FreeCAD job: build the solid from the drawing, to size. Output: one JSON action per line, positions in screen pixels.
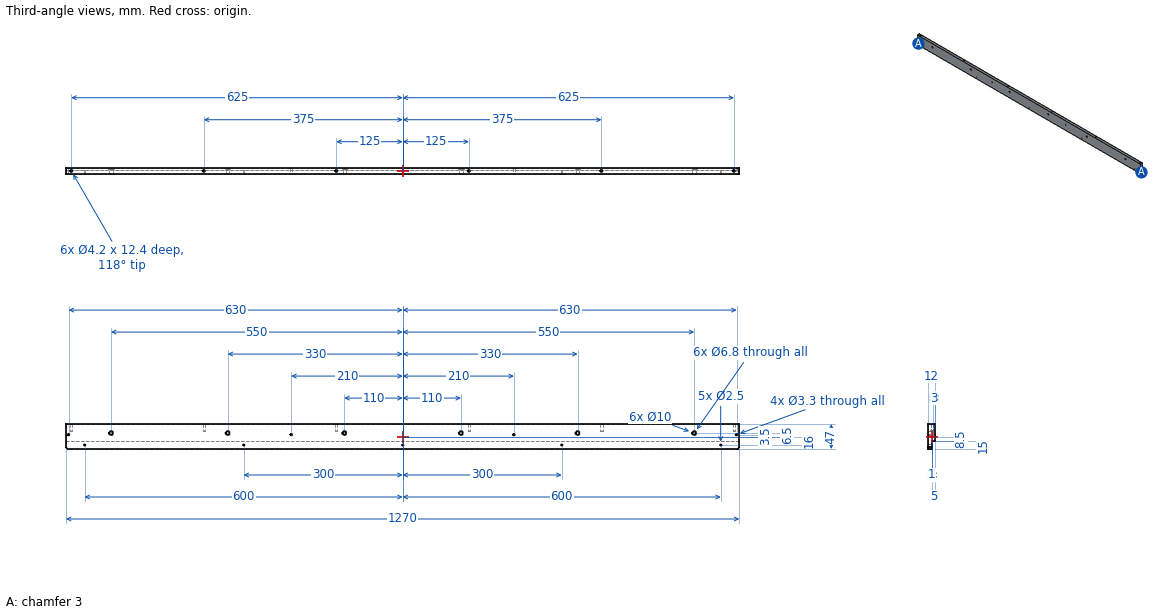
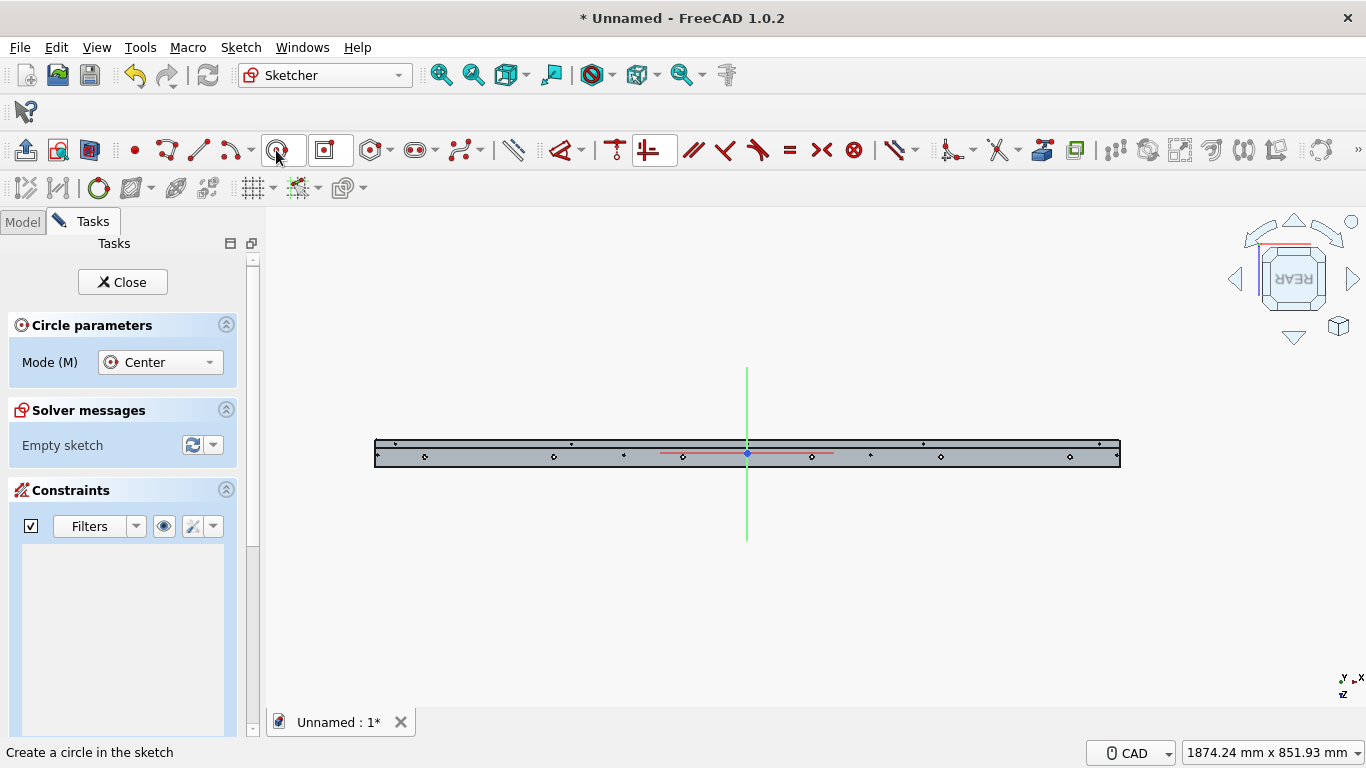
{"action": "scroll", "coordinate": [1070, 457], "scroll_direction": "up", "scroll_amount": 11}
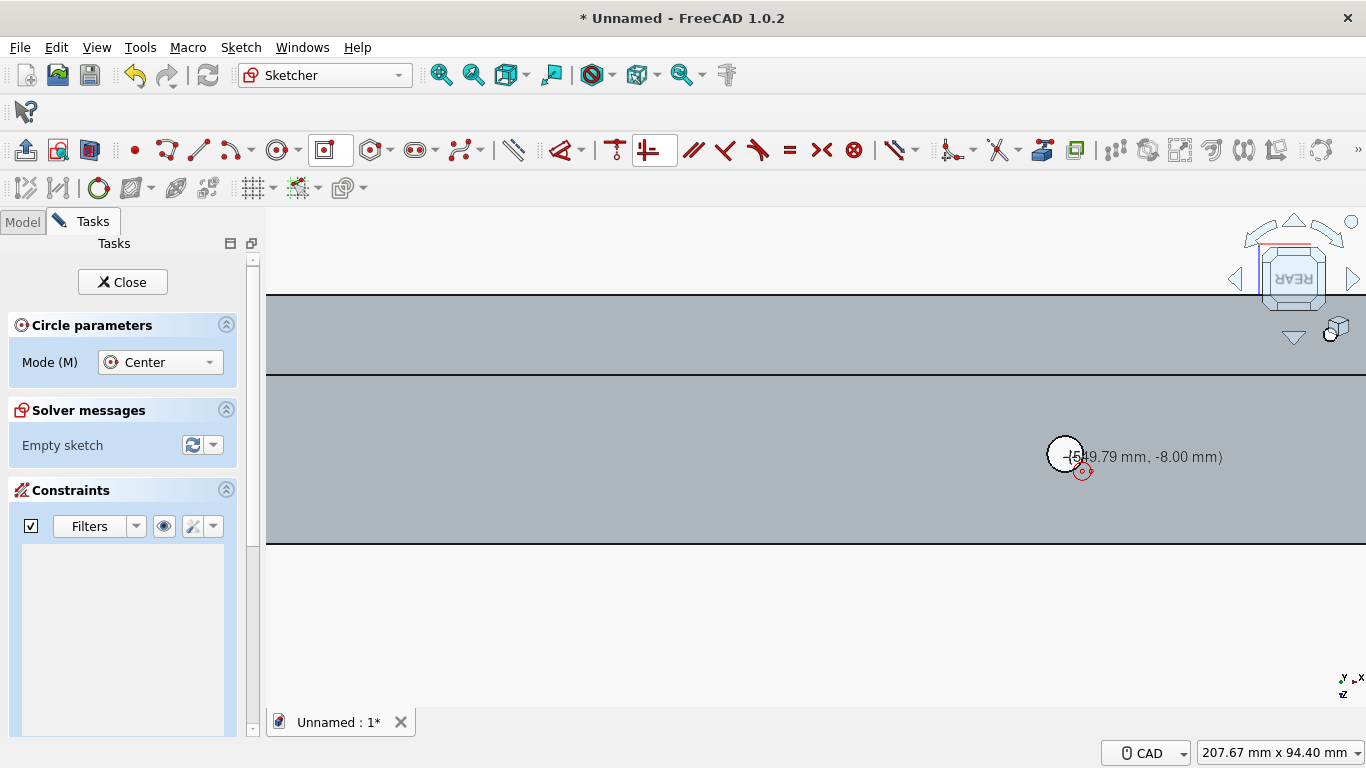
{"action": "left_click", "coordinate": [1065, 454]}
{"action": "mouse_move", "coordinate": [1084, 435]}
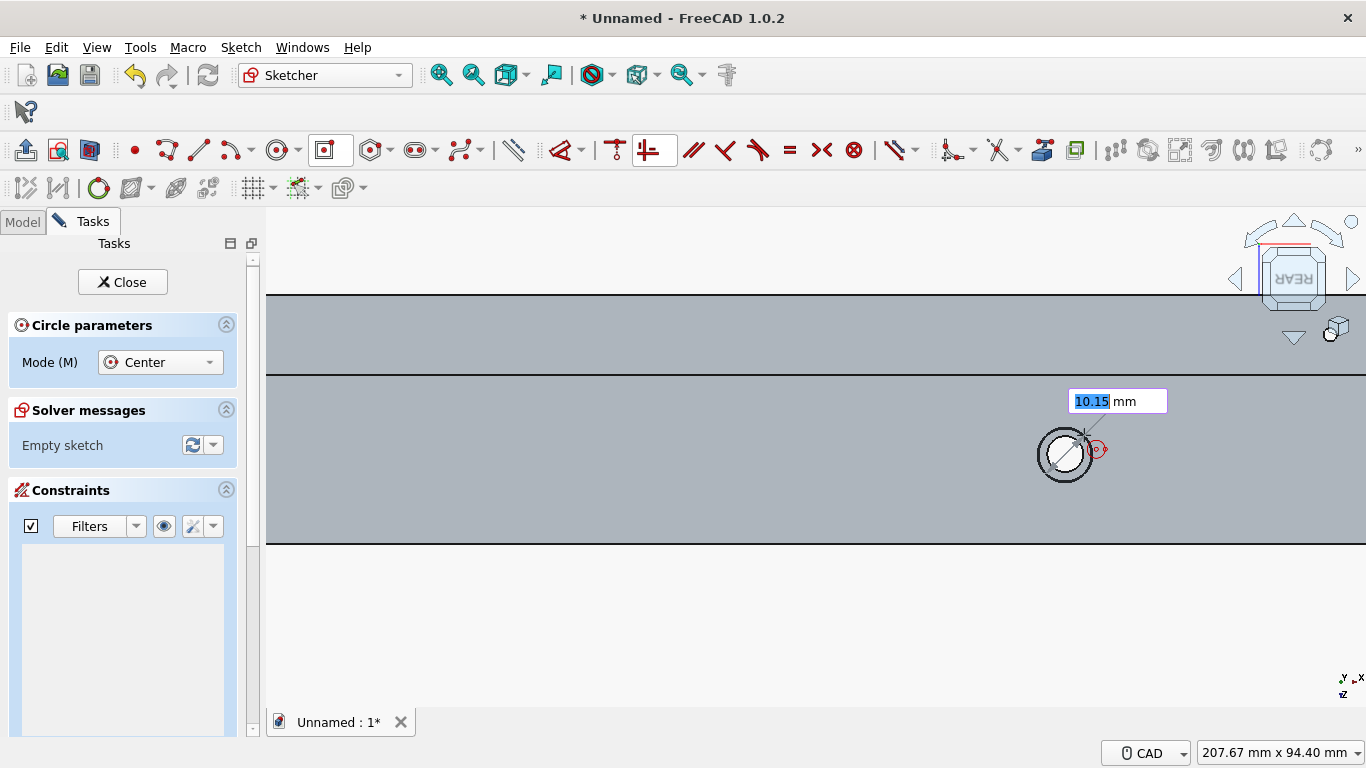
{"action": "type", "text": "10"}
{"action": "key", "text": "Return"}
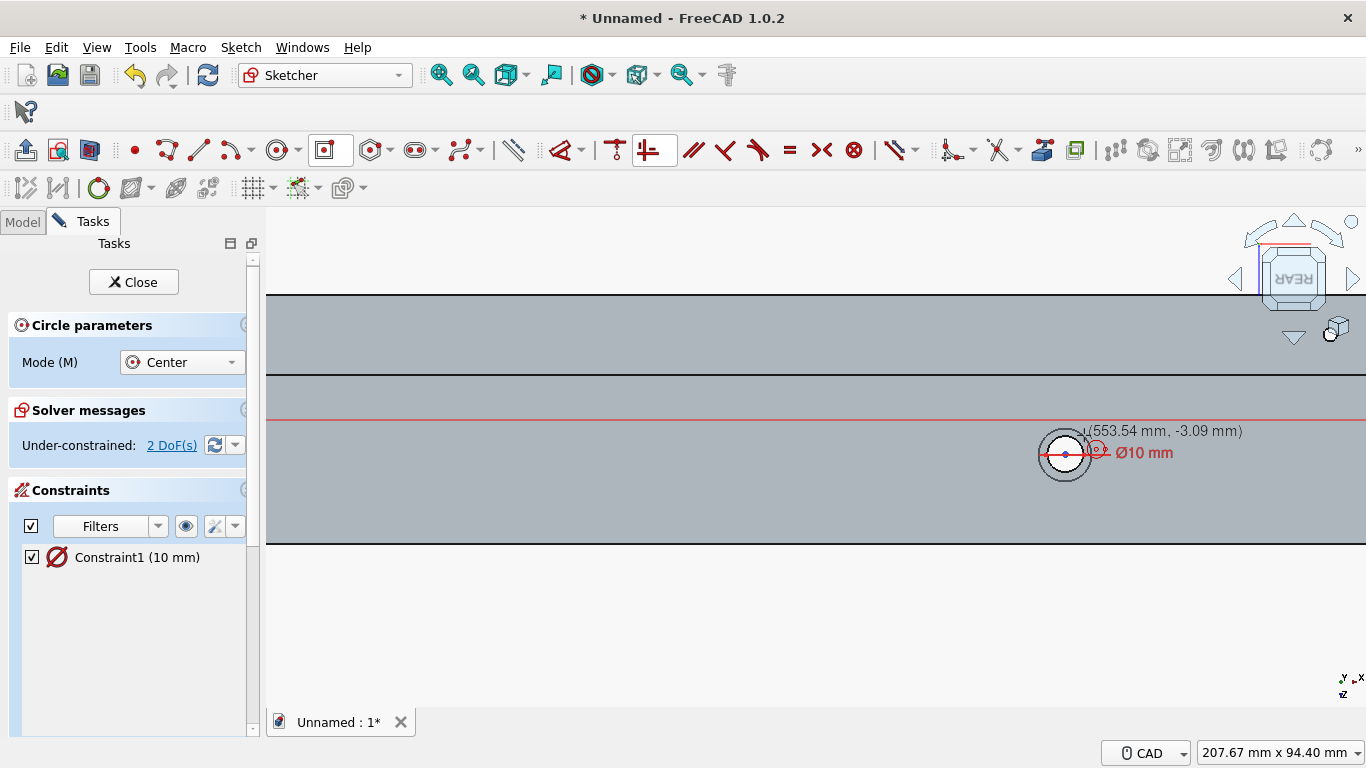
{"action": "scroll", "coordinate": [1071, 458], "scroll_direction": "down", "scroll_amount": 11}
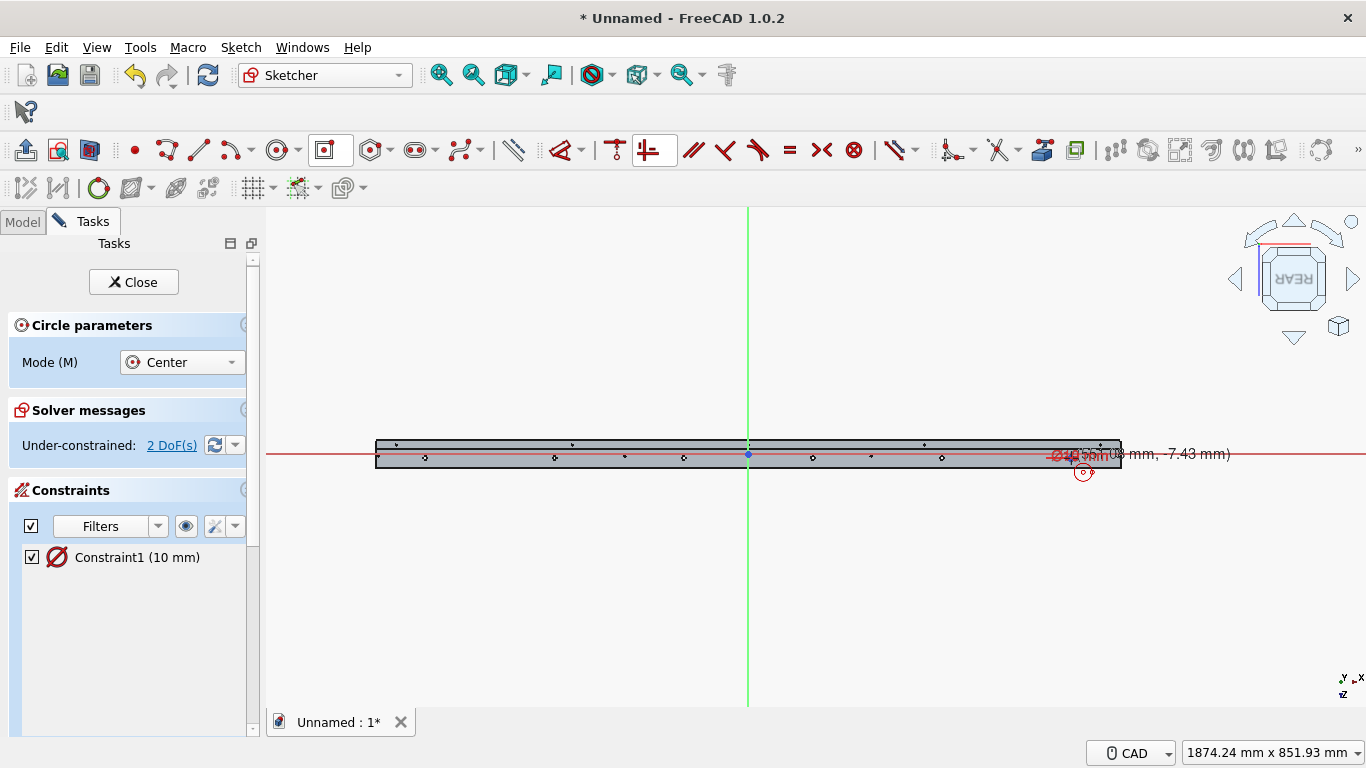
{"action": "scroll", "coordinate": [942, 458], "scroll_direction": "up", "scroll_amount": 11}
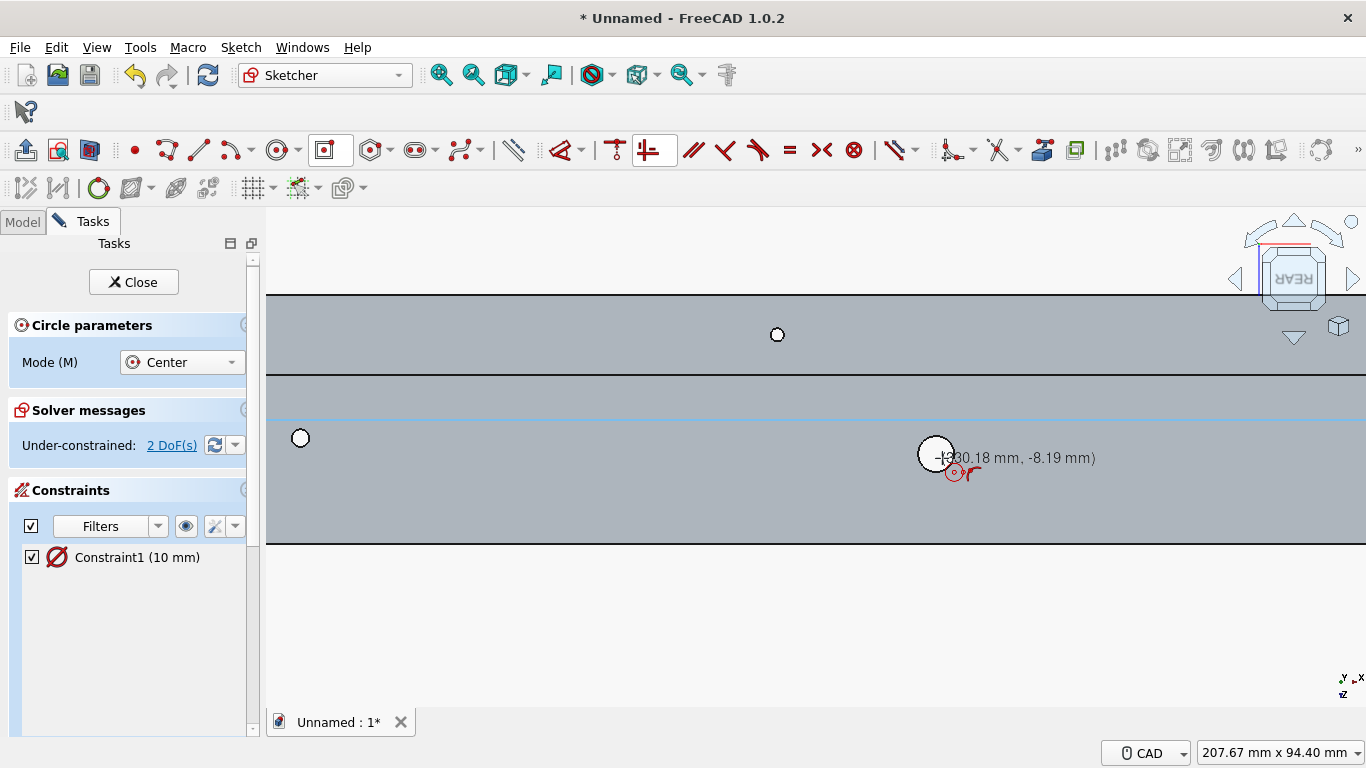
{"action": "left_click", "coordinate": [936, 454]}
{"action": "mouse_move", "coordinate": [955, 435]}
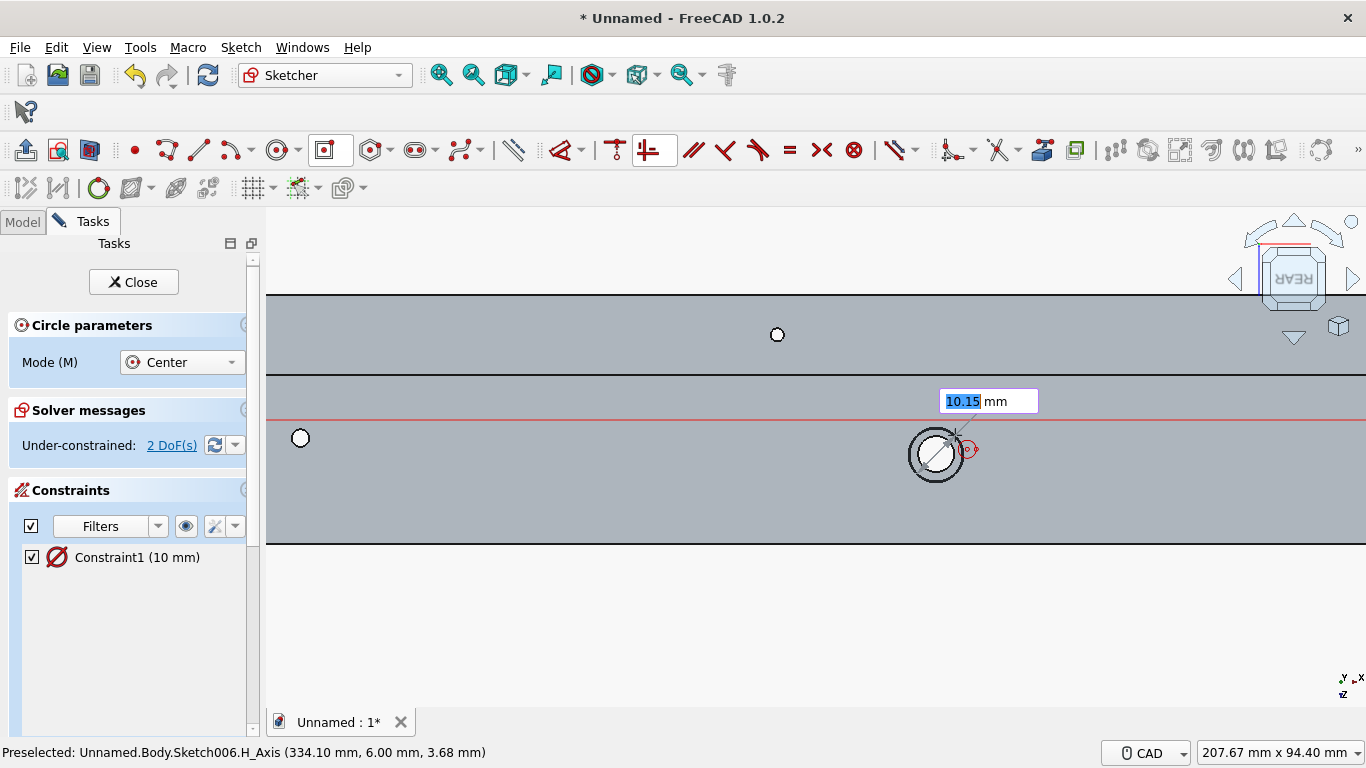
{"action": "type", "text": "10"}
{"action": "key", "text": "Return"}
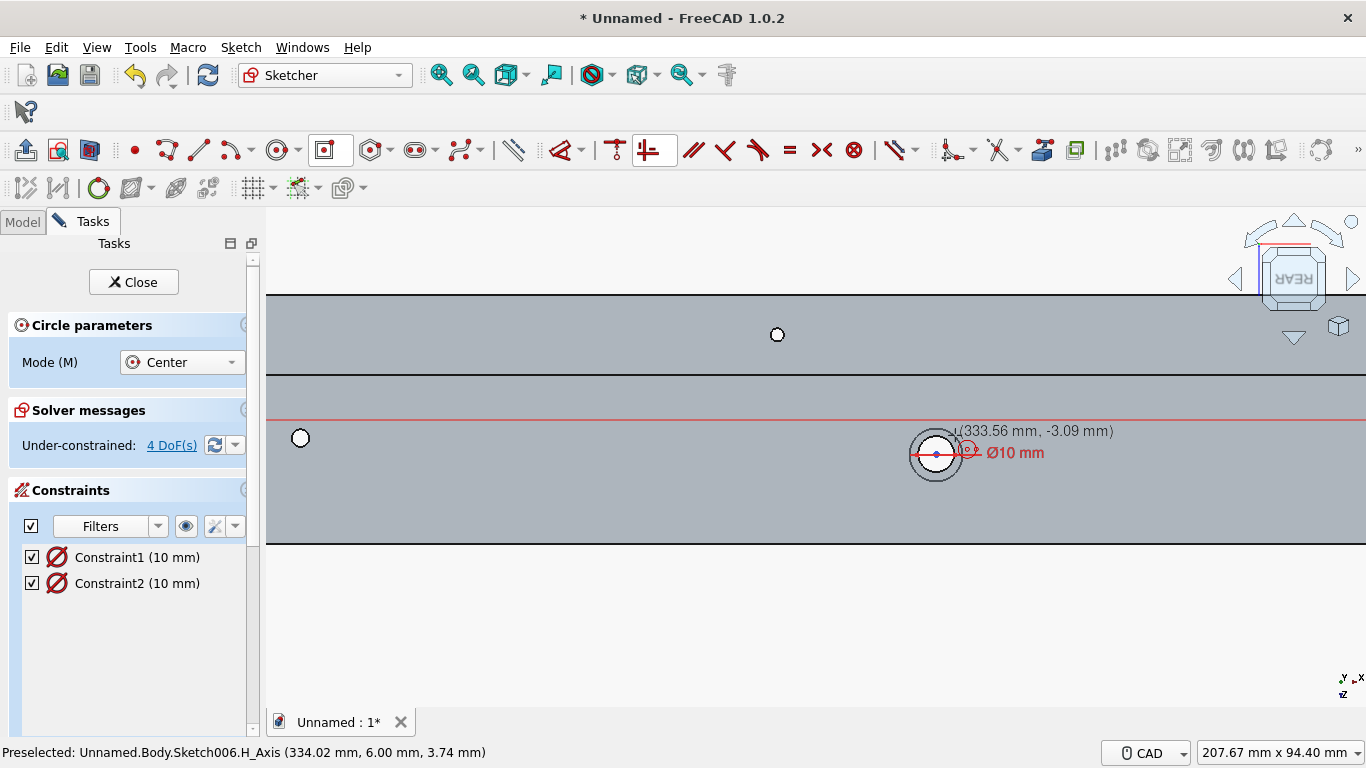
{"action": "scroll", "coordinate": [942, 458], "scroll_direction": "down", "scroll_amount": 11}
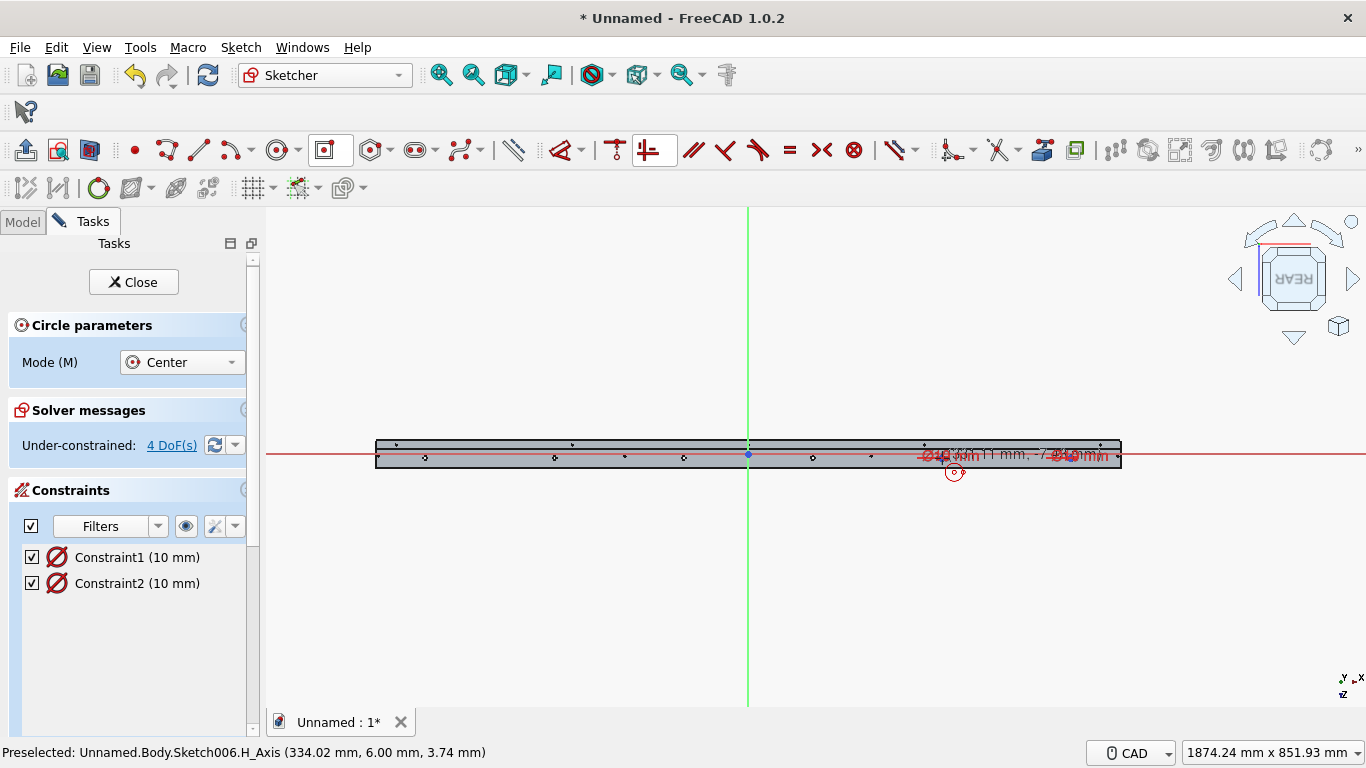
{"action": "scroll", "coordinate": [813, 458], "scroll_direction": "up", "scroll_amount": 11}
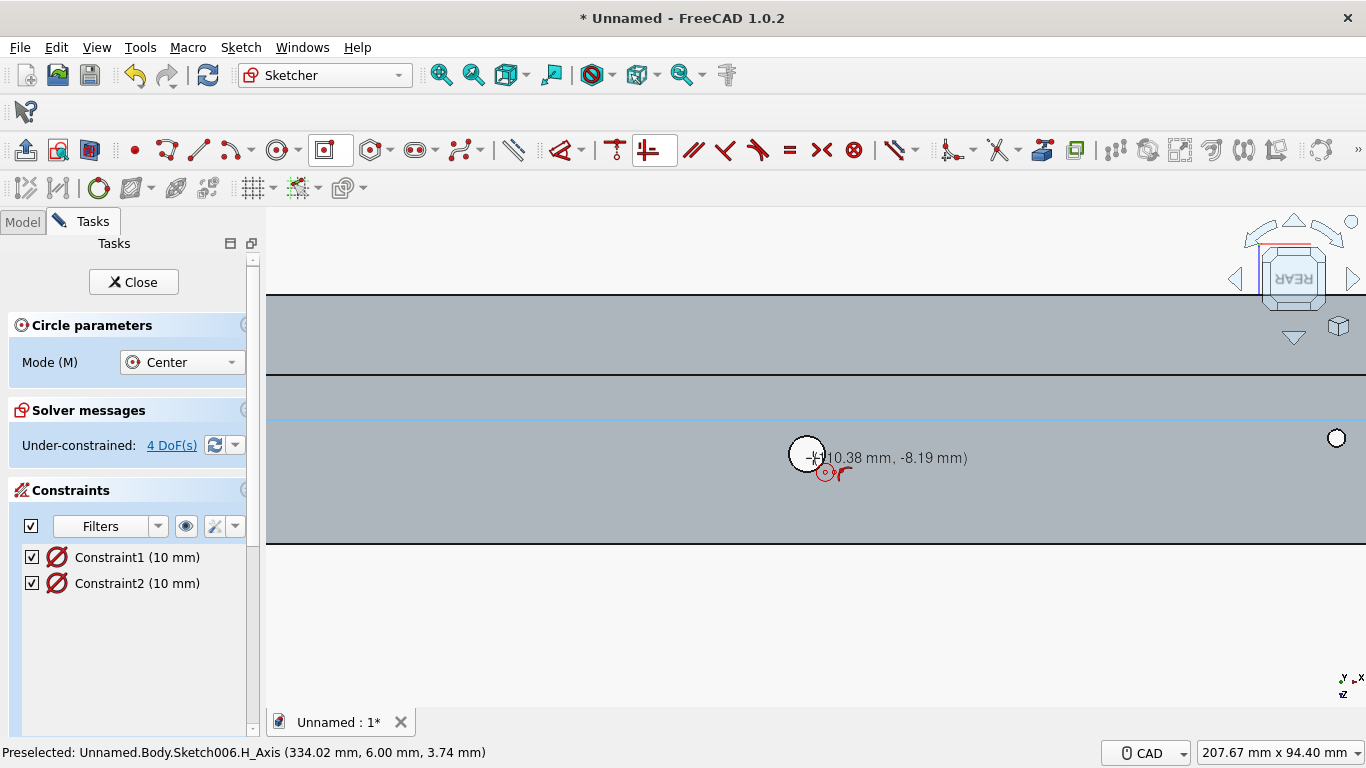
{"action": "left_click", "coordinate": [807, 454]}
{"action": "mouse_move", "coordinate": [826, 435]}